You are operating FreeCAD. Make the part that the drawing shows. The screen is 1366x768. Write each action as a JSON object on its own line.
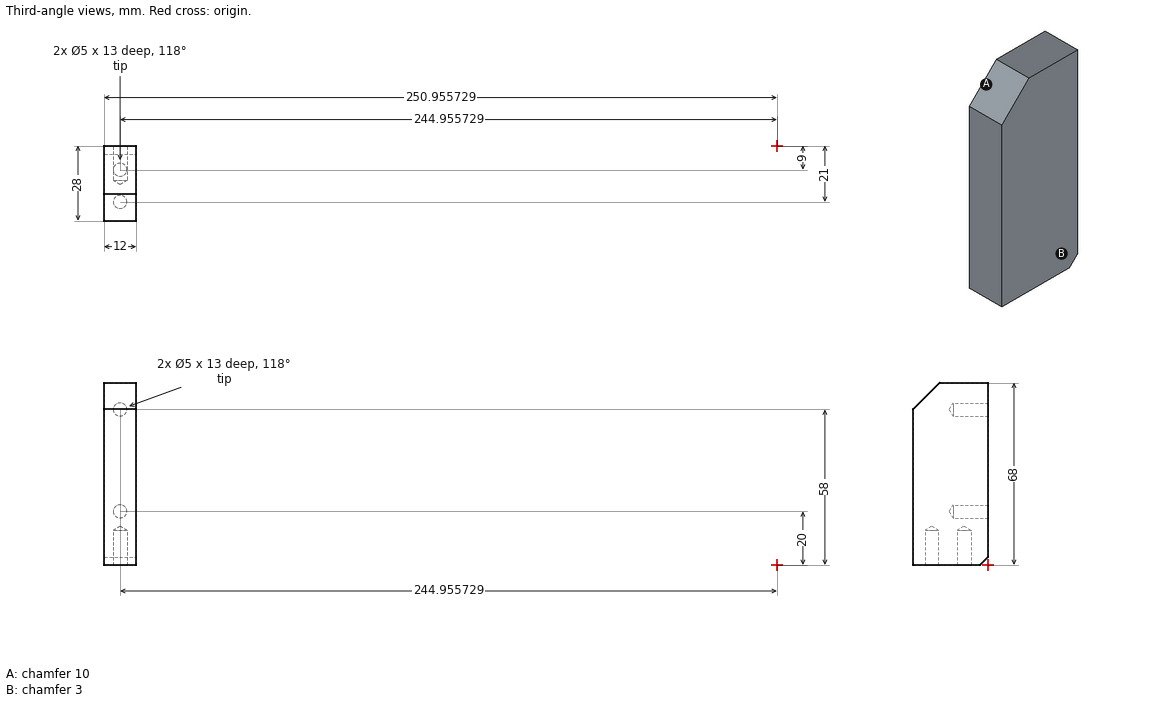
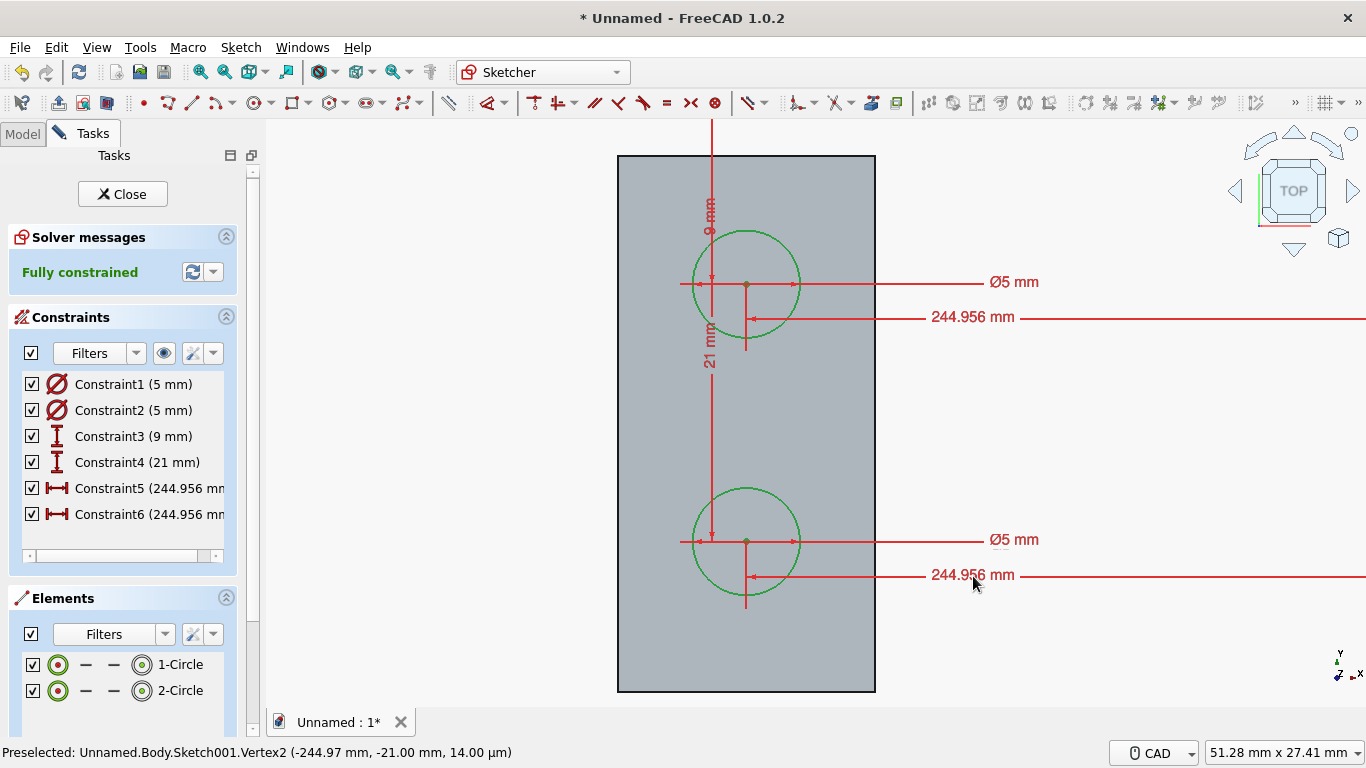
{"action": "left_click", "coordinate": [123, 194]}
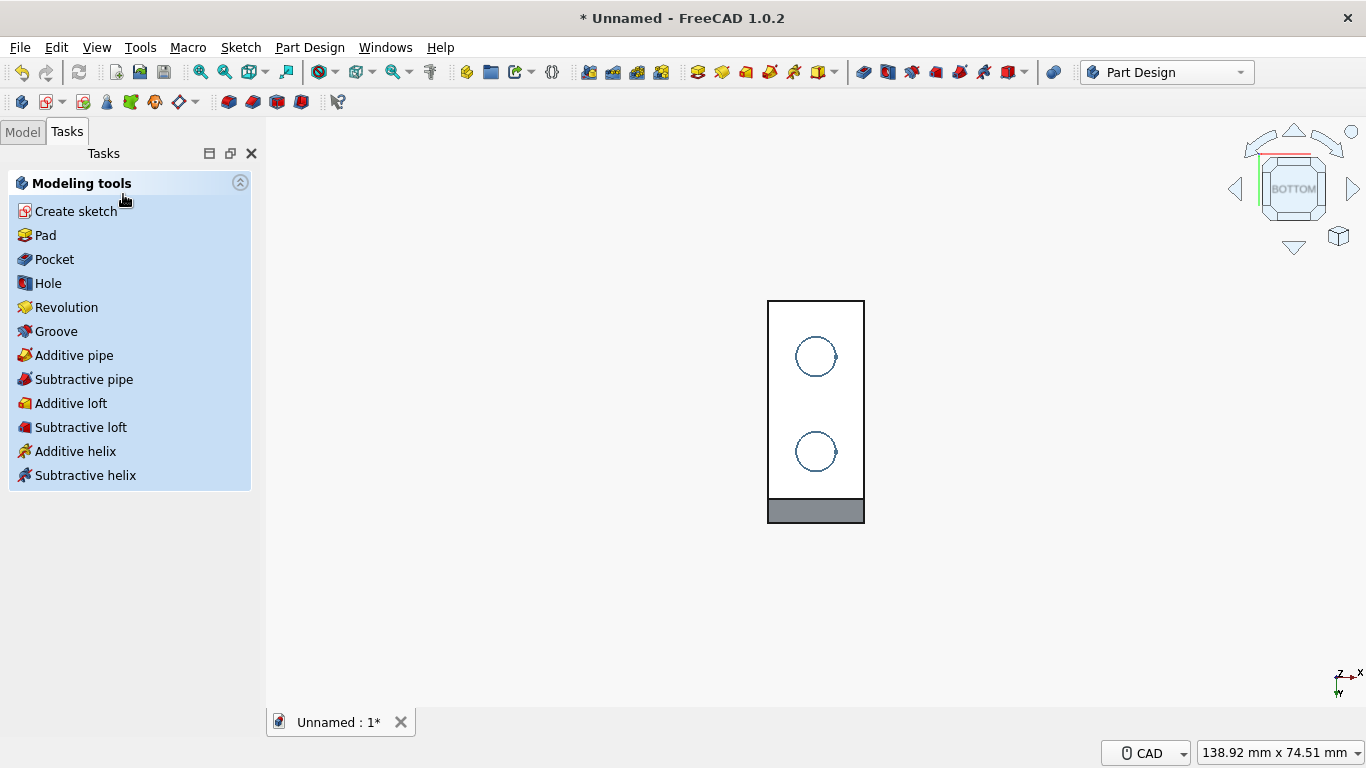
{"action": "left_click", "coordinate": [888, 72]}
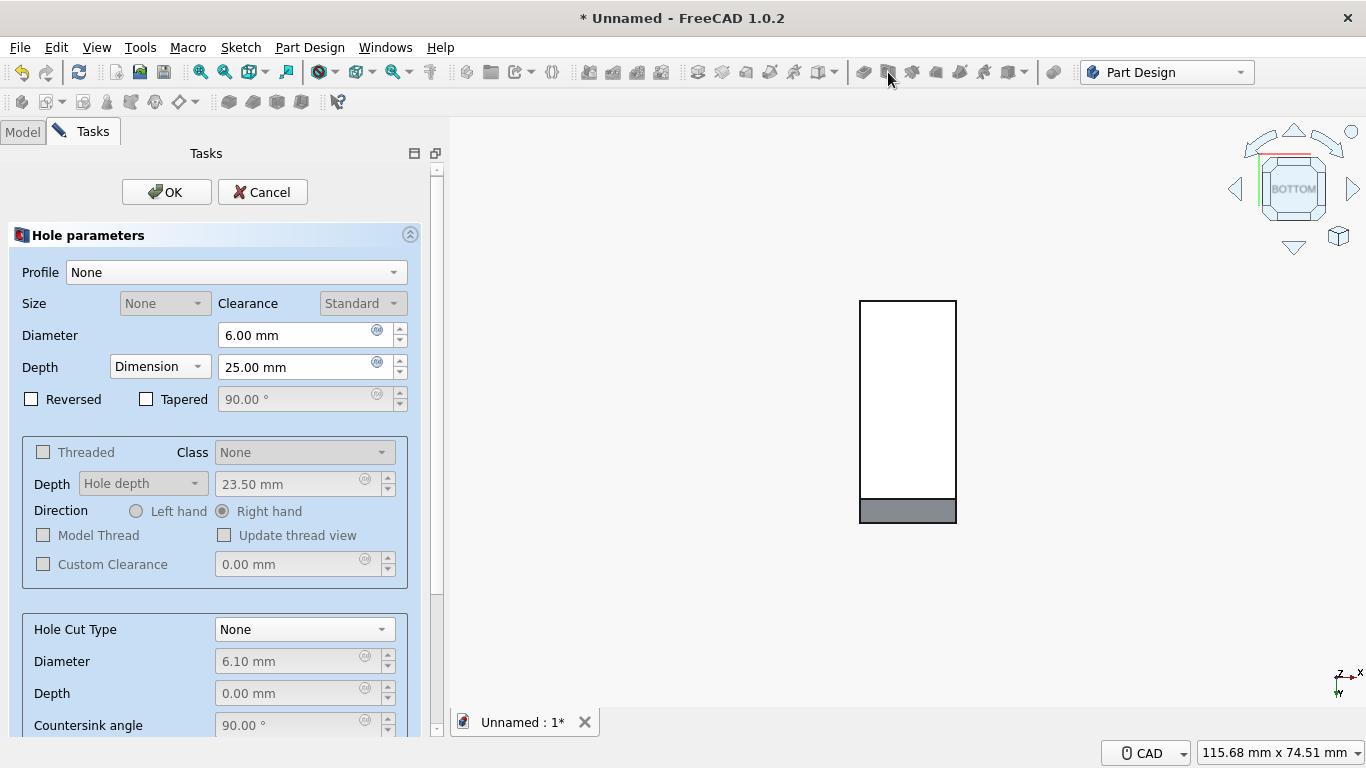
{"action": "triple_click", "coordinate": [305, 335]}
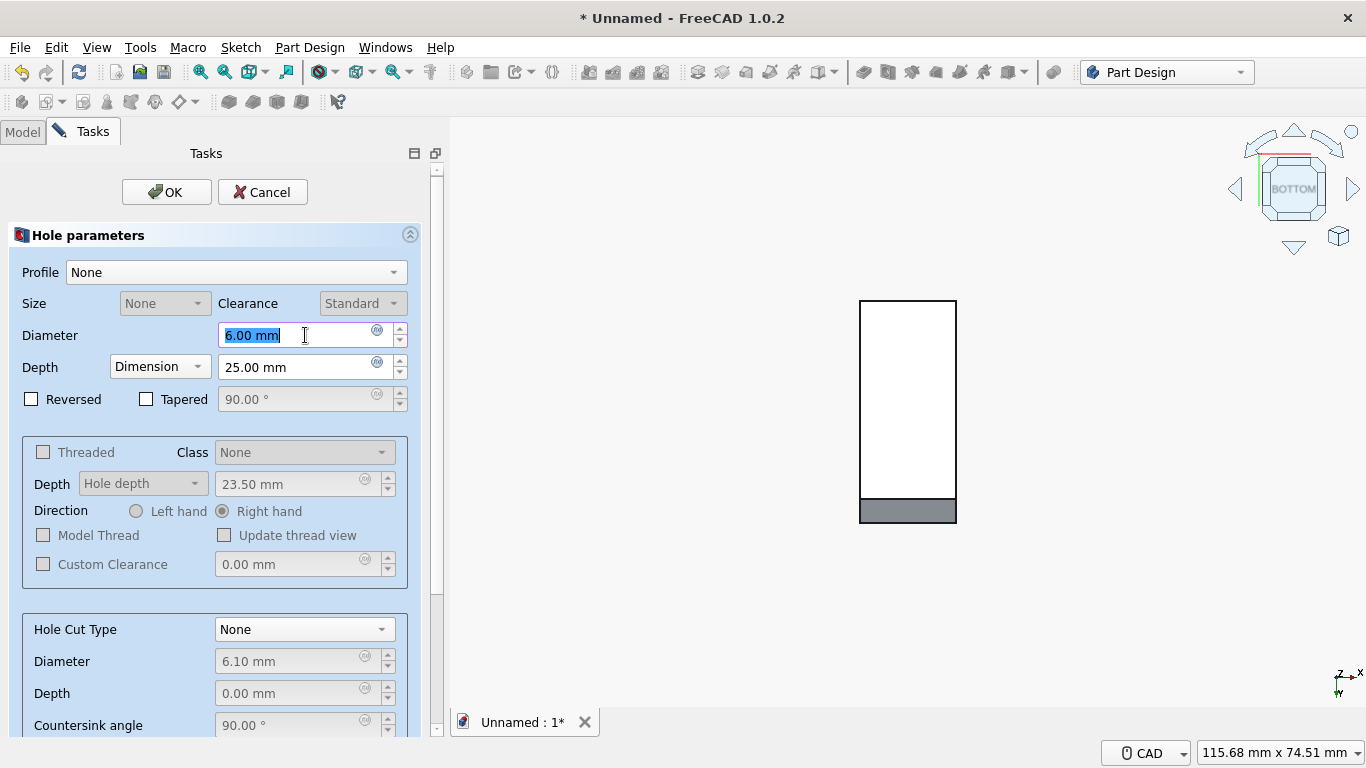
{"action": "type", "text": "5"}
{"action": "key", "text": "Tab"}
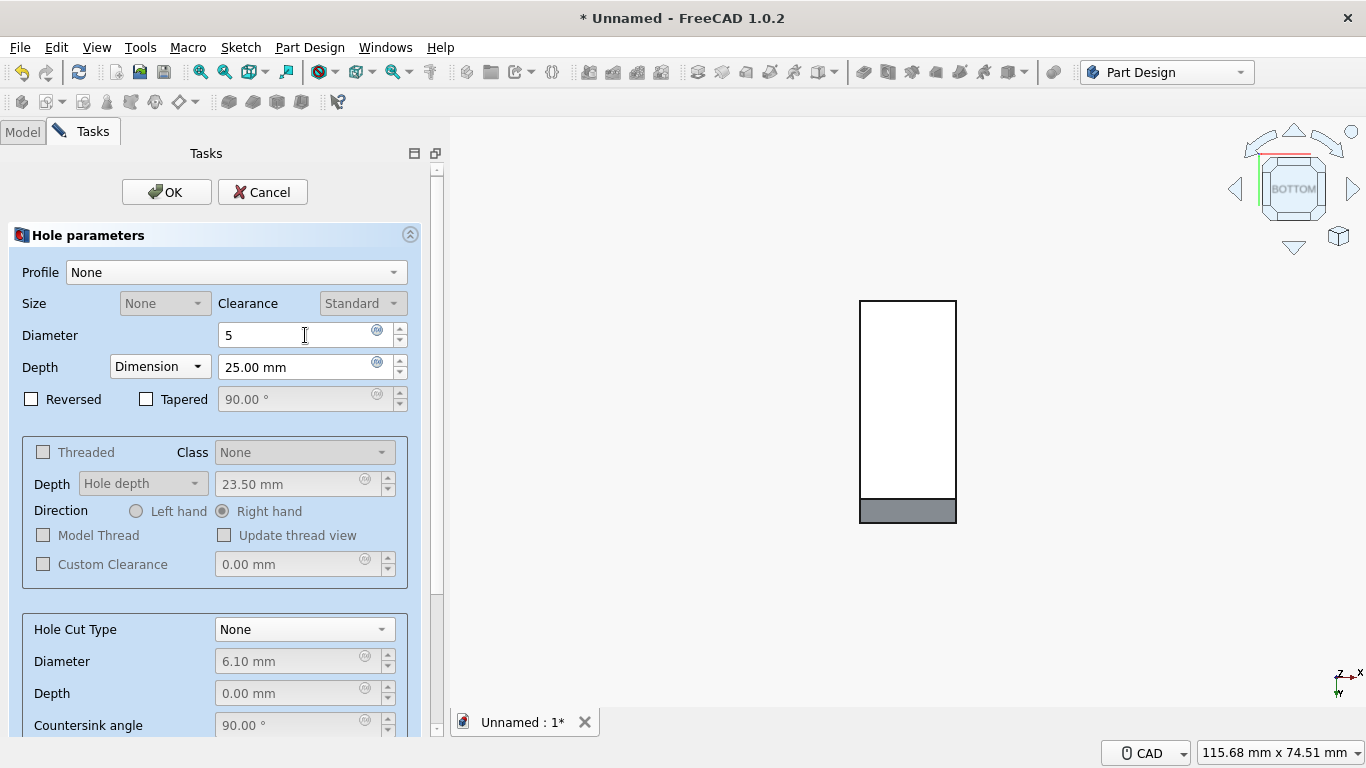
{"action": "triple_click", "coordinate": [305, 367]}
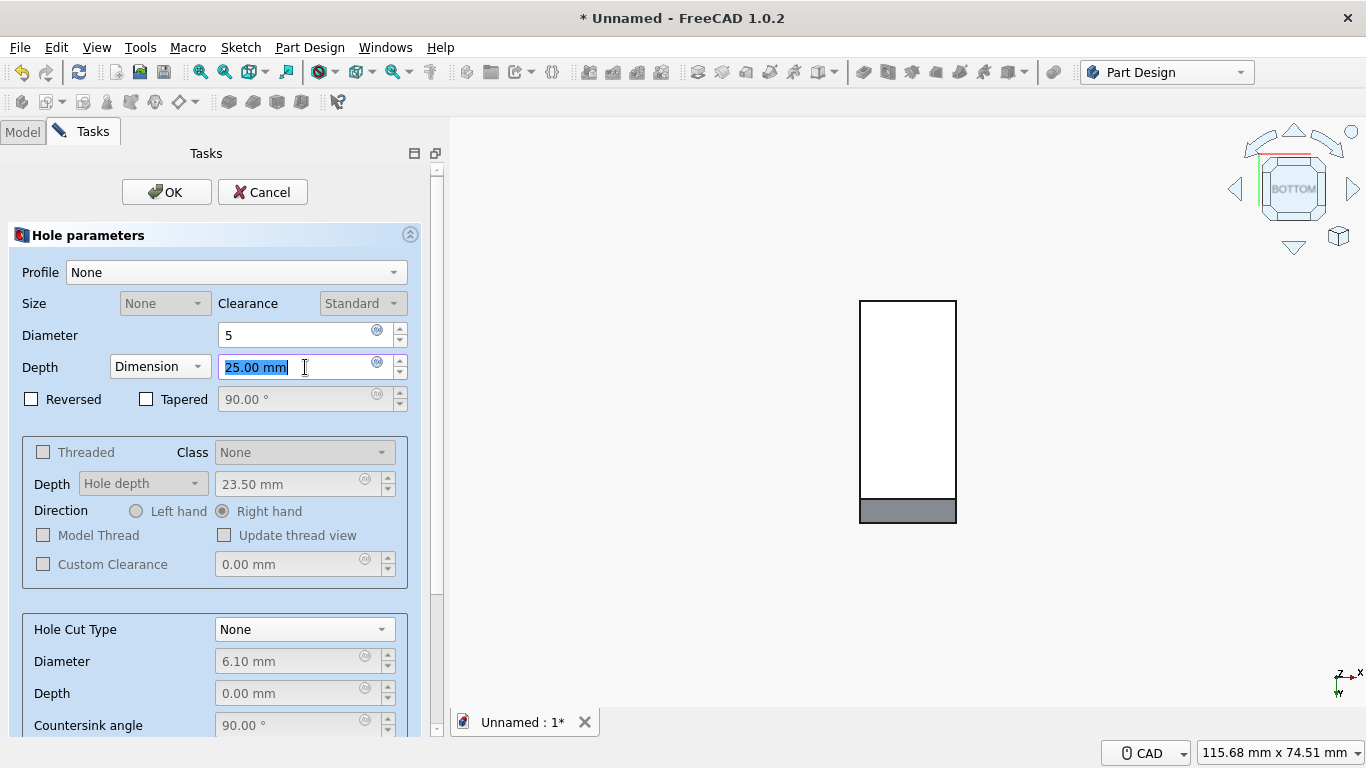
{"action": "type", "text": "13"}
{"action": "key", "text": "Tab"}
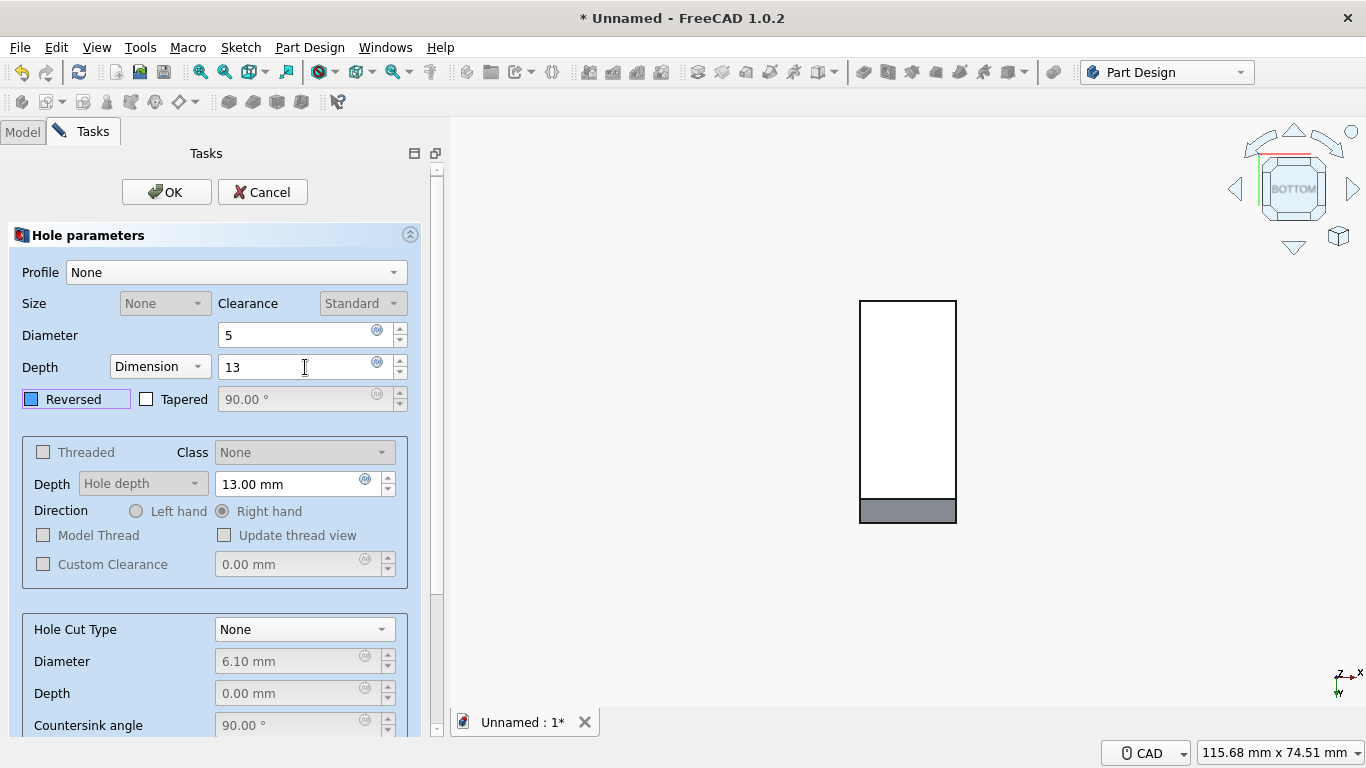
{"action": "left_click", "coordinate": [30, 399]}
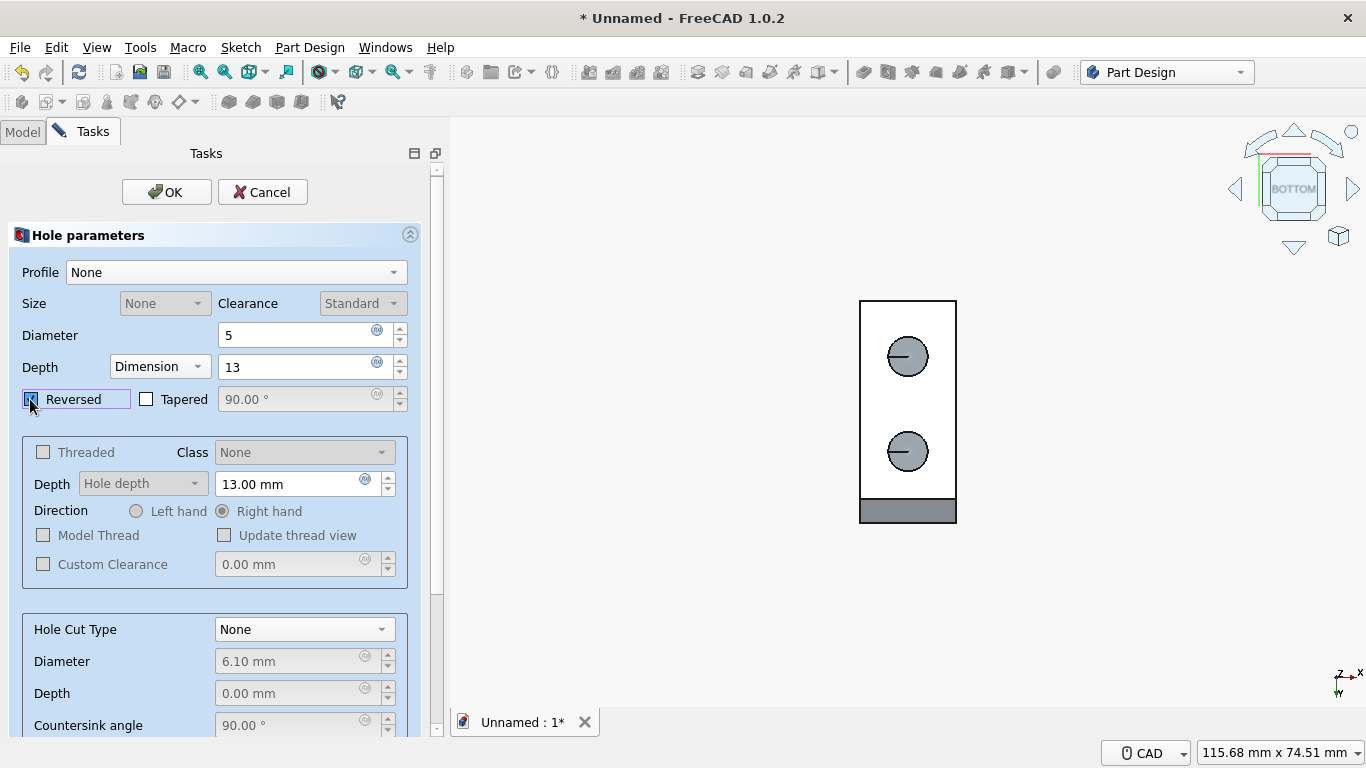
{"action": "left_click", "coordinate": [167, 192]}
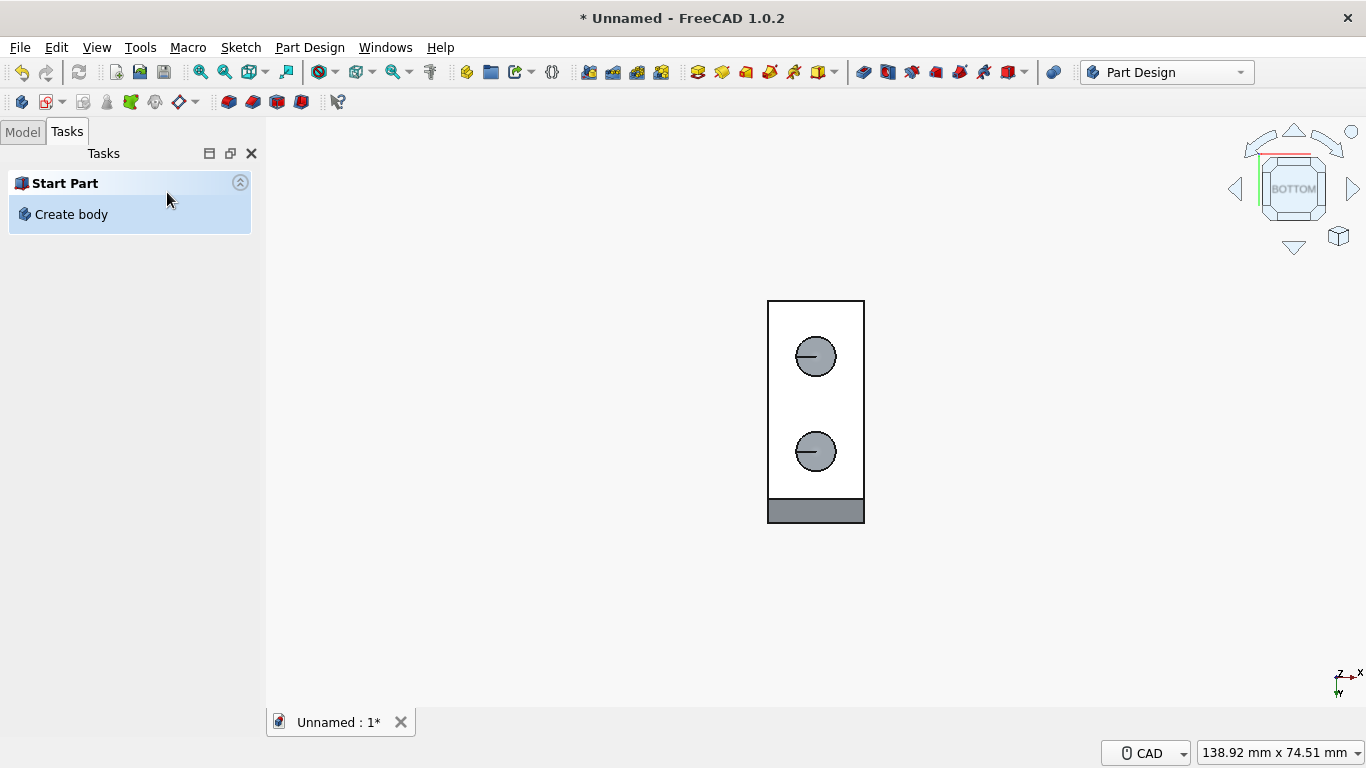
{"action": "key", "text": "v f"}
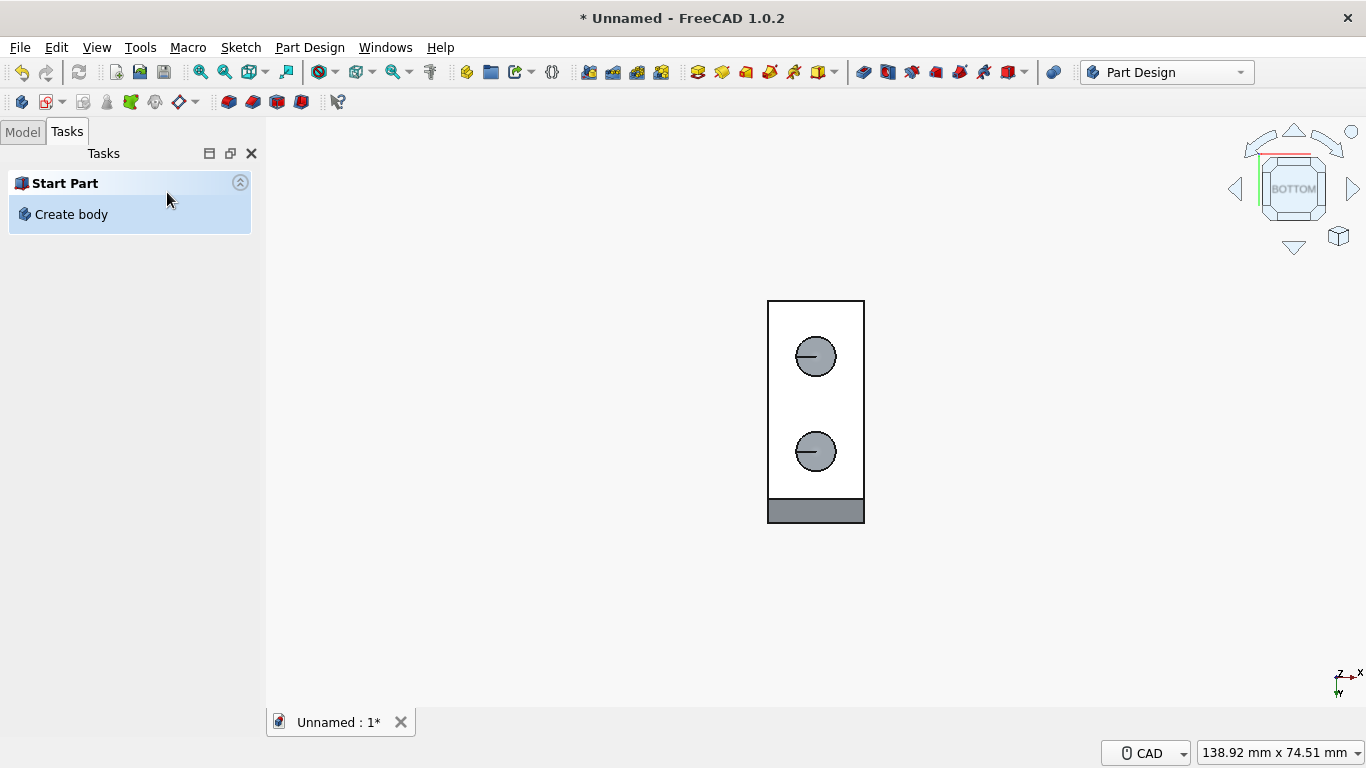
{"action": "left_click", "coordinate": [46, 102]}